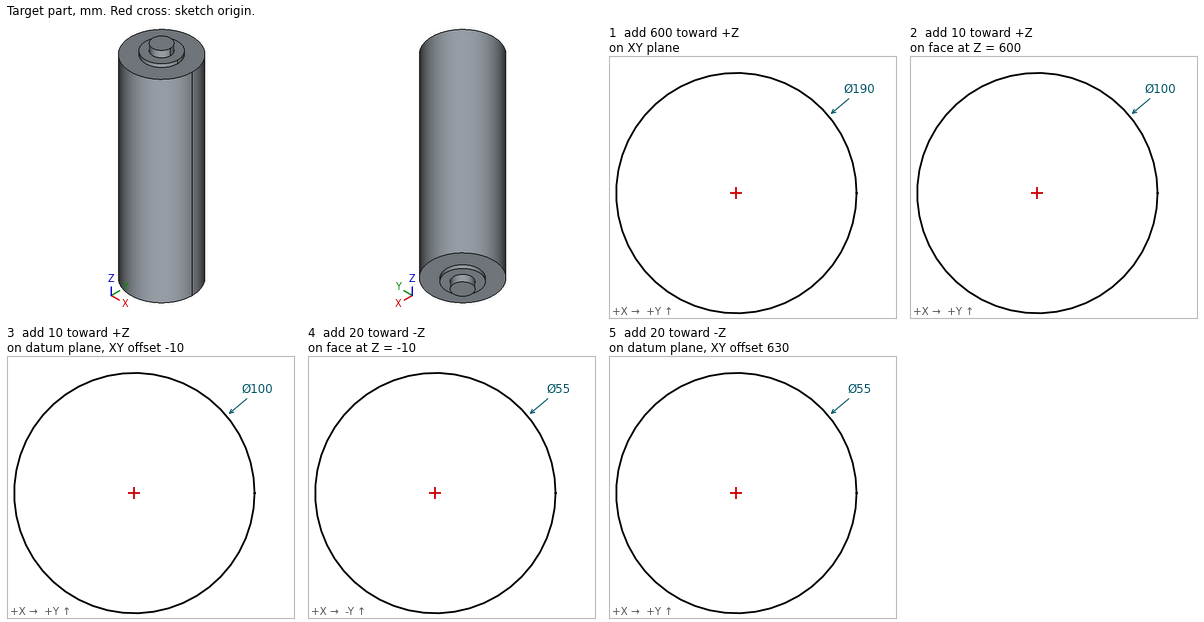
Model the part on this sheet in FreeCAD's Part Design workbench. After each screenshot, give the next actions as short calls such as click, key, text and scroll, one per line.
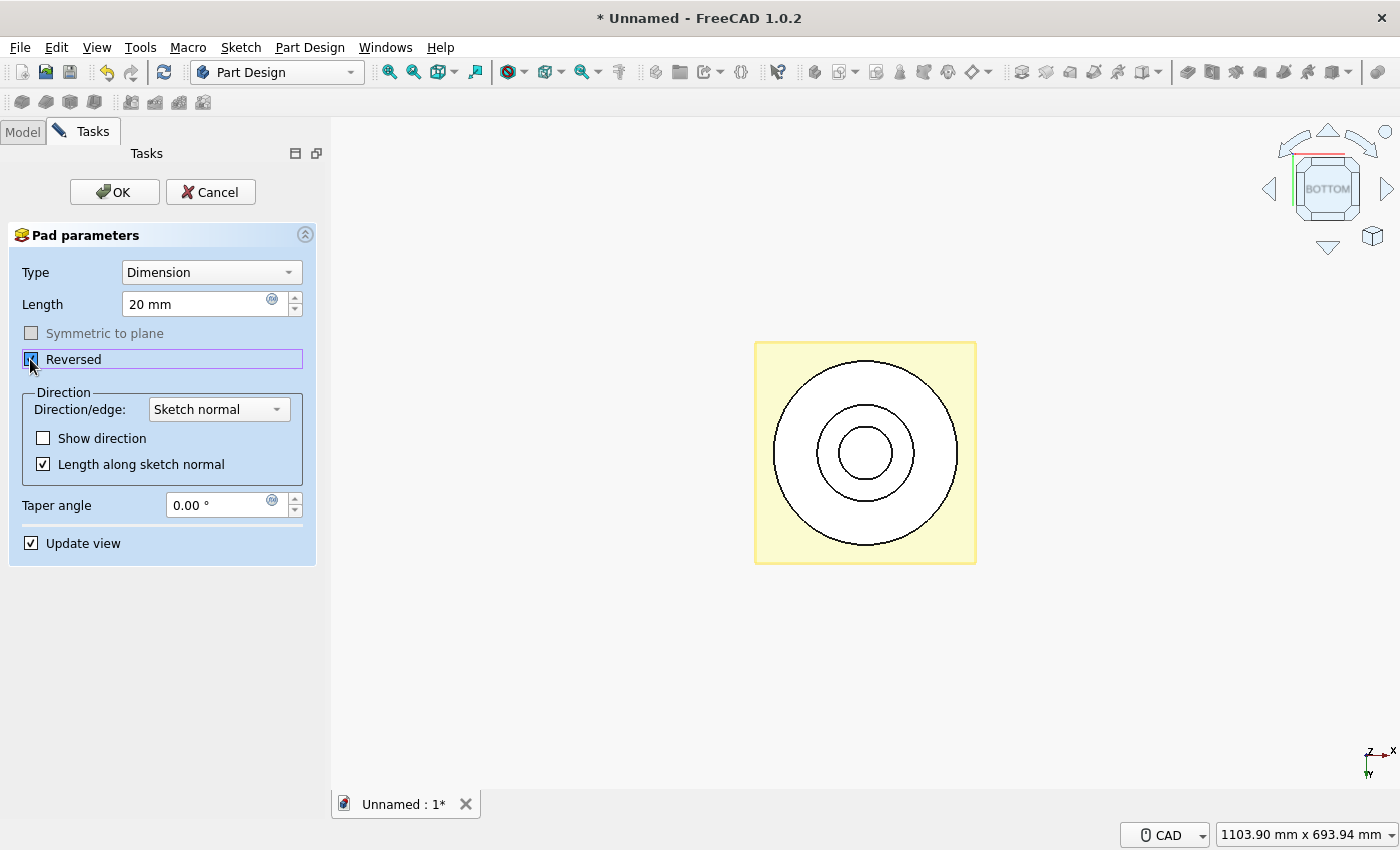
click(115, 192)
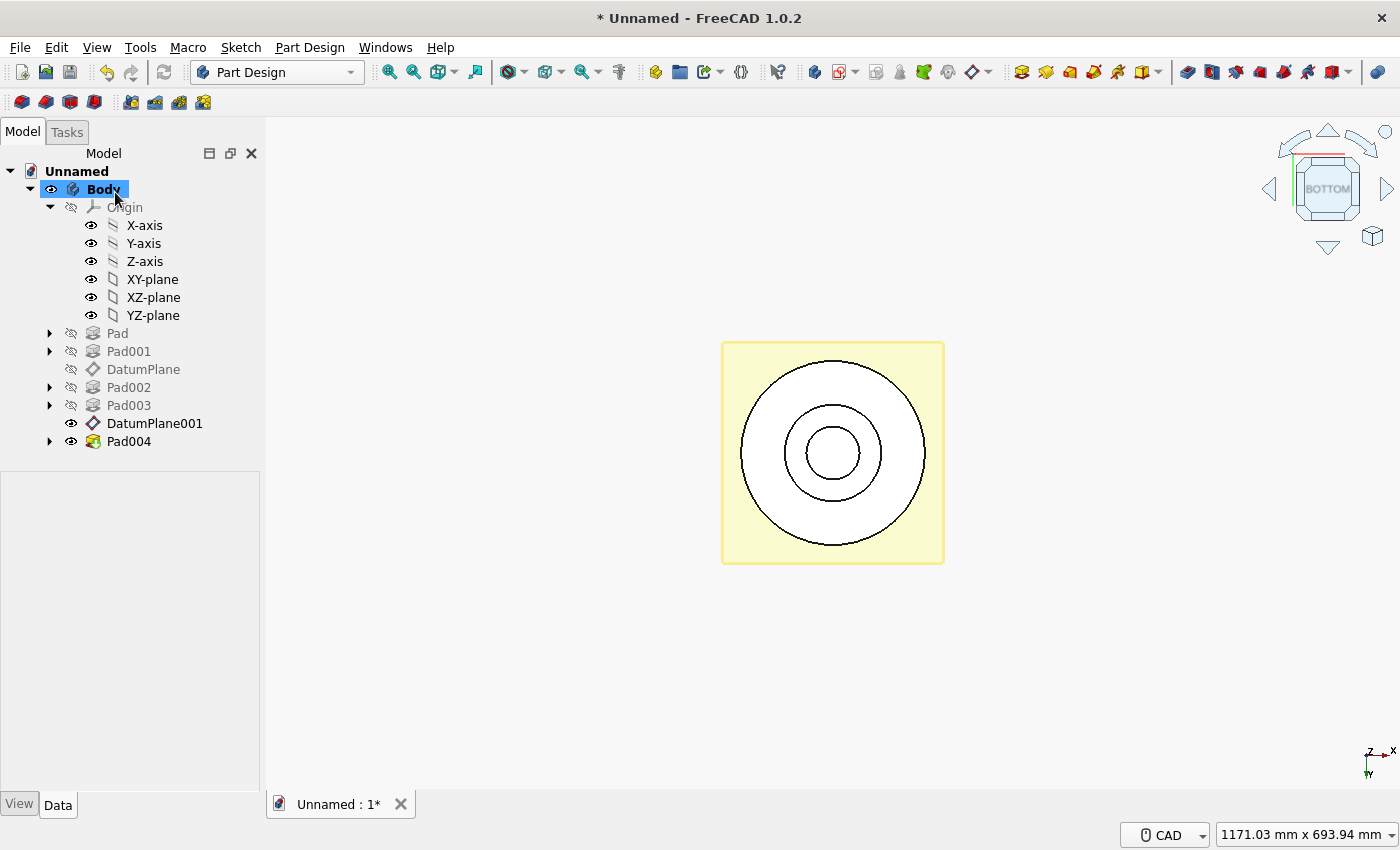
click(116, 423)
key(space)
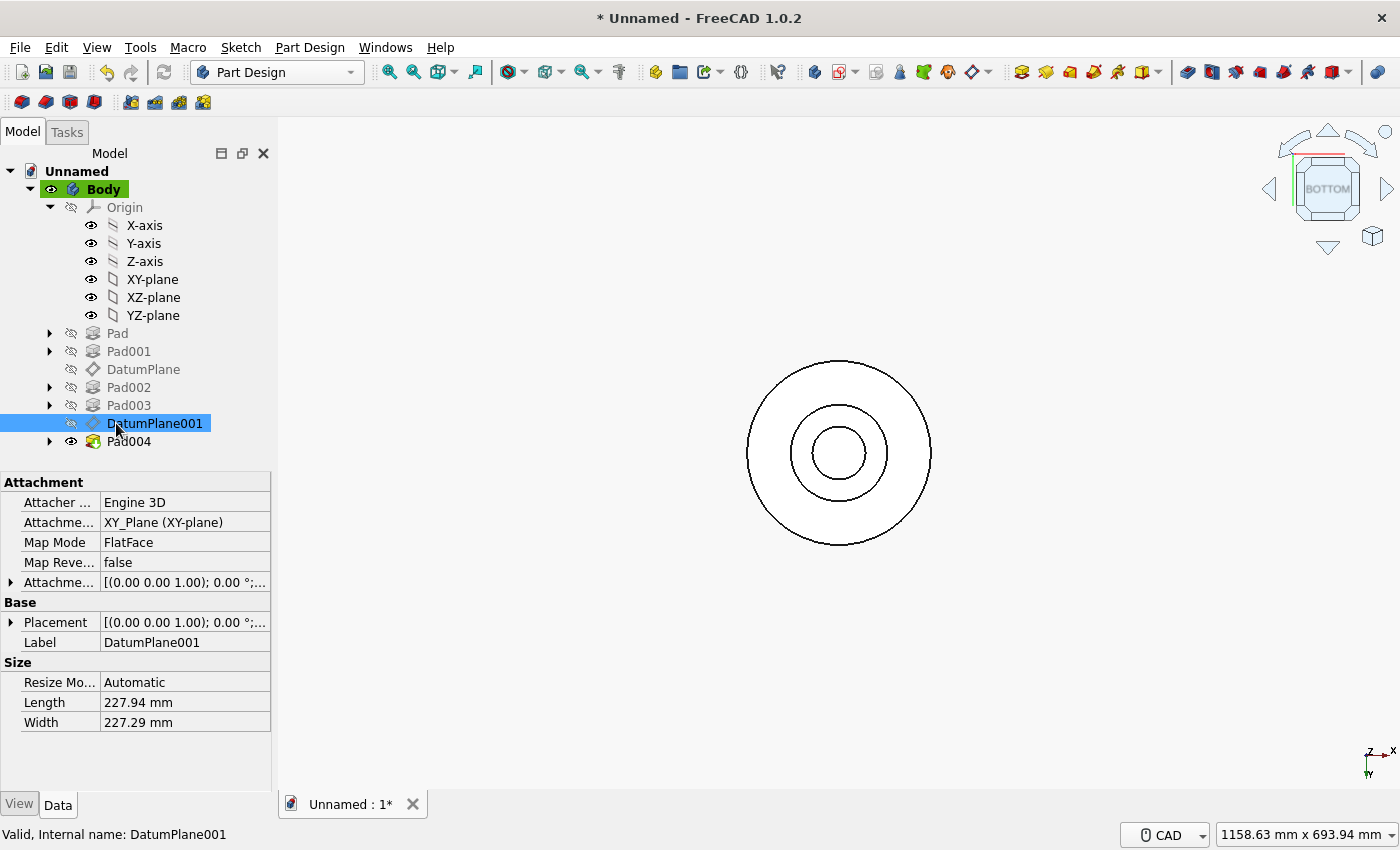
key(0)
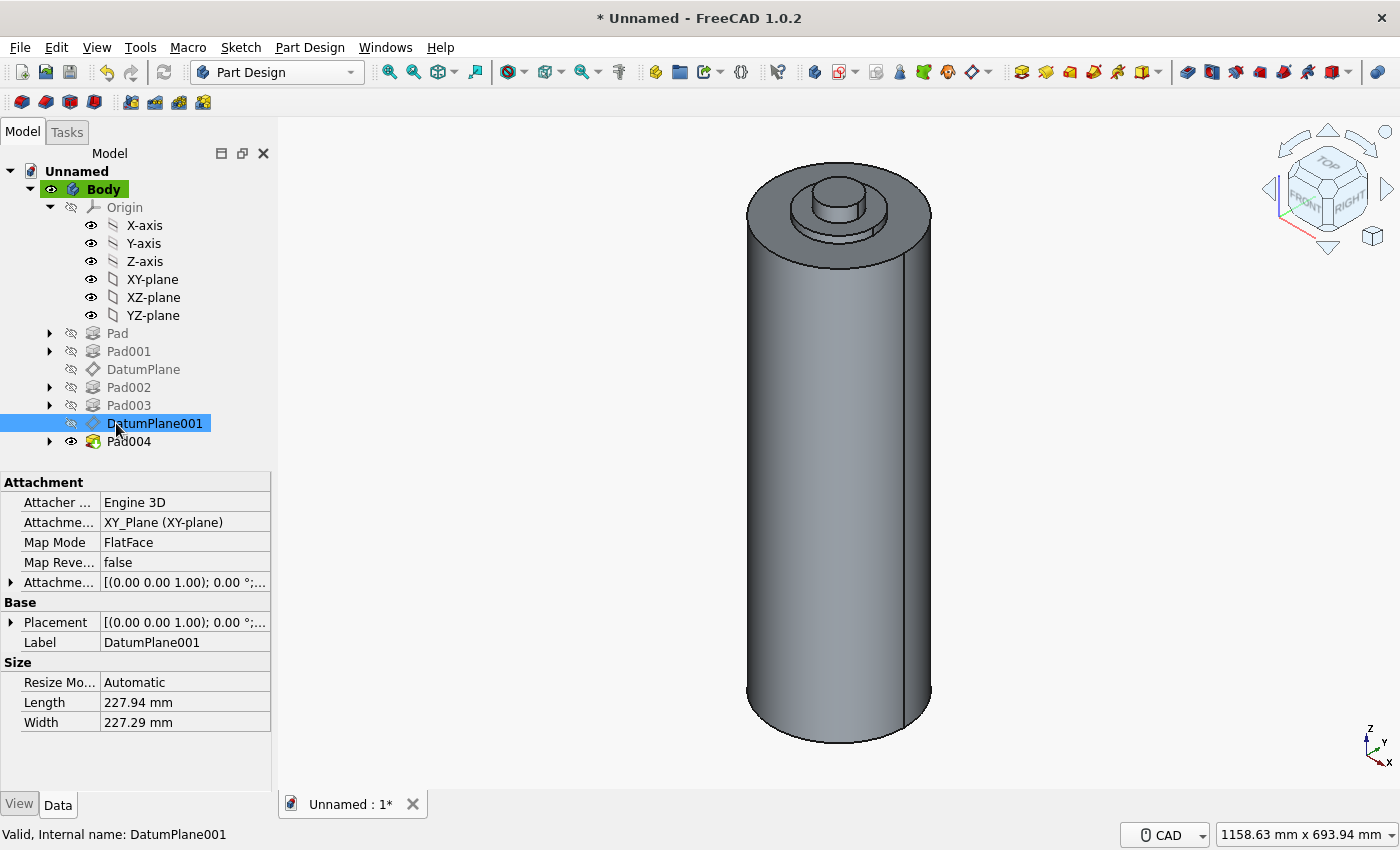
key(v)
key(f)